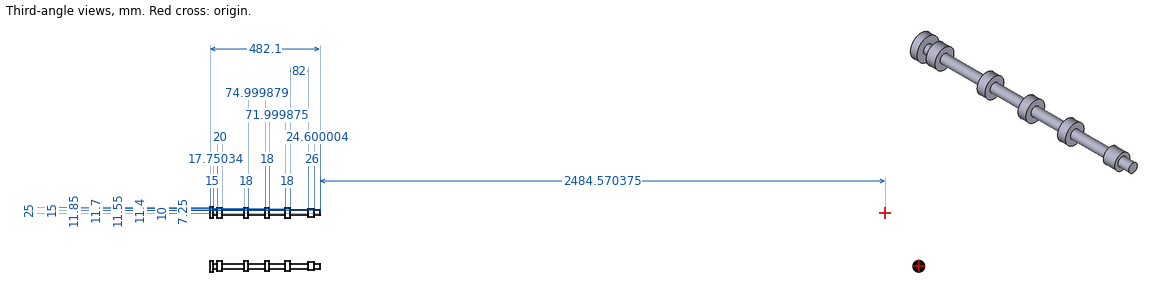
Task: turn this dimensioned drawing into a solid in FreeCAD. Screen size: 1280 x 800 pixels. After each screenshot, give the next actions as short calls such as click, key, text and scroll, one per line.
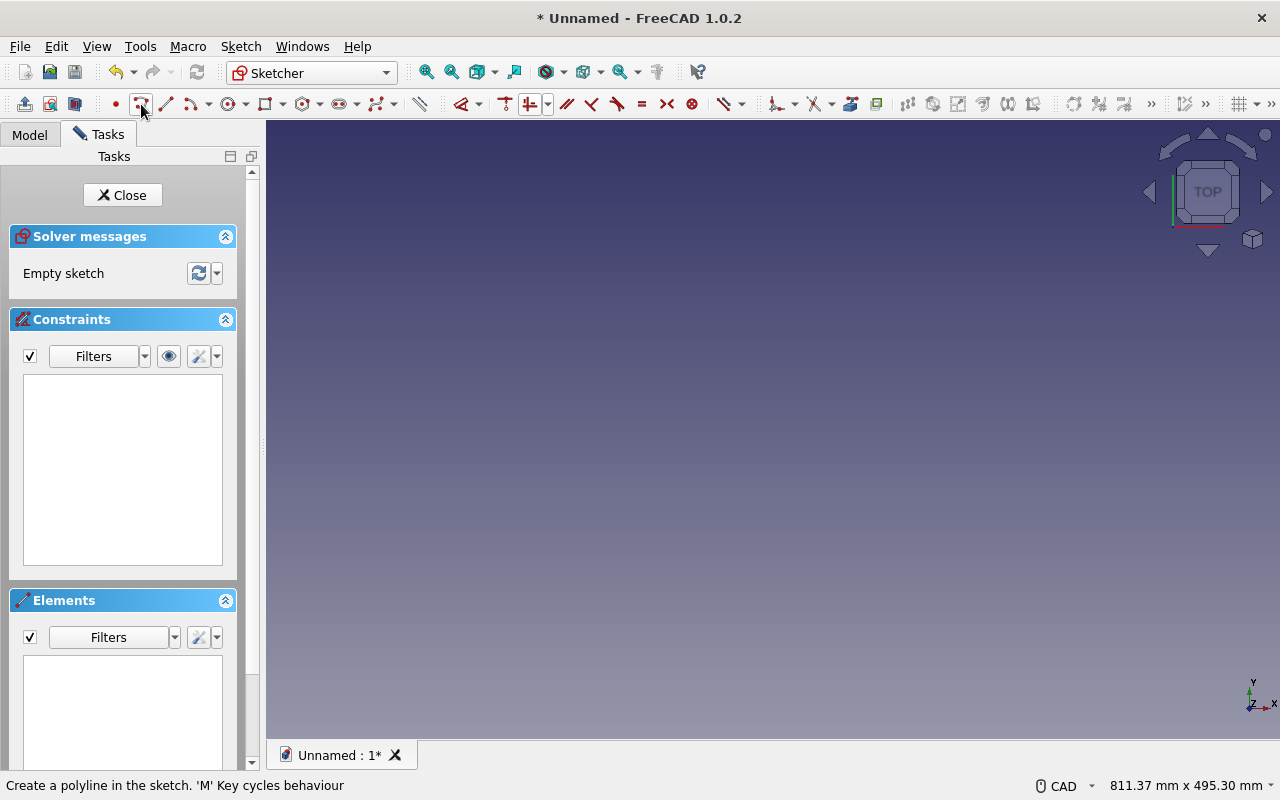
click(995, 430)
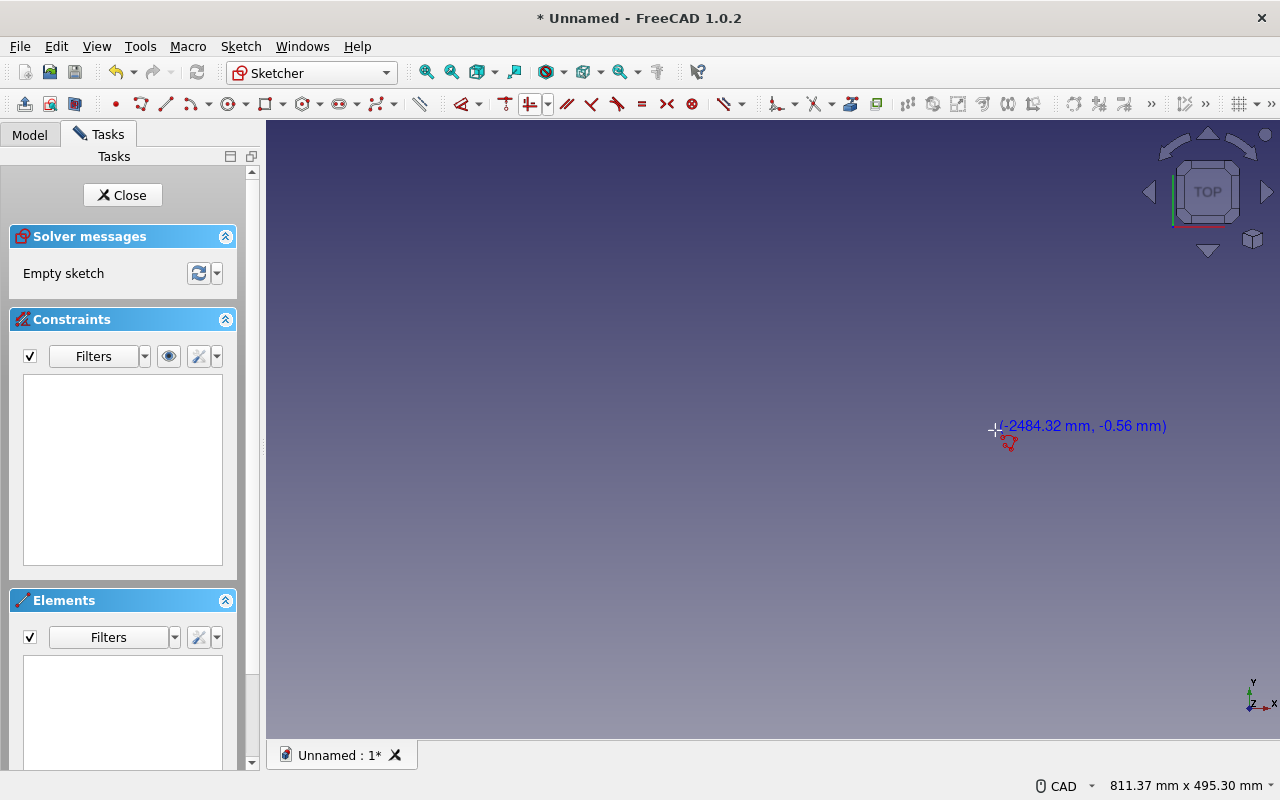
scroll(995, 418, up, 2)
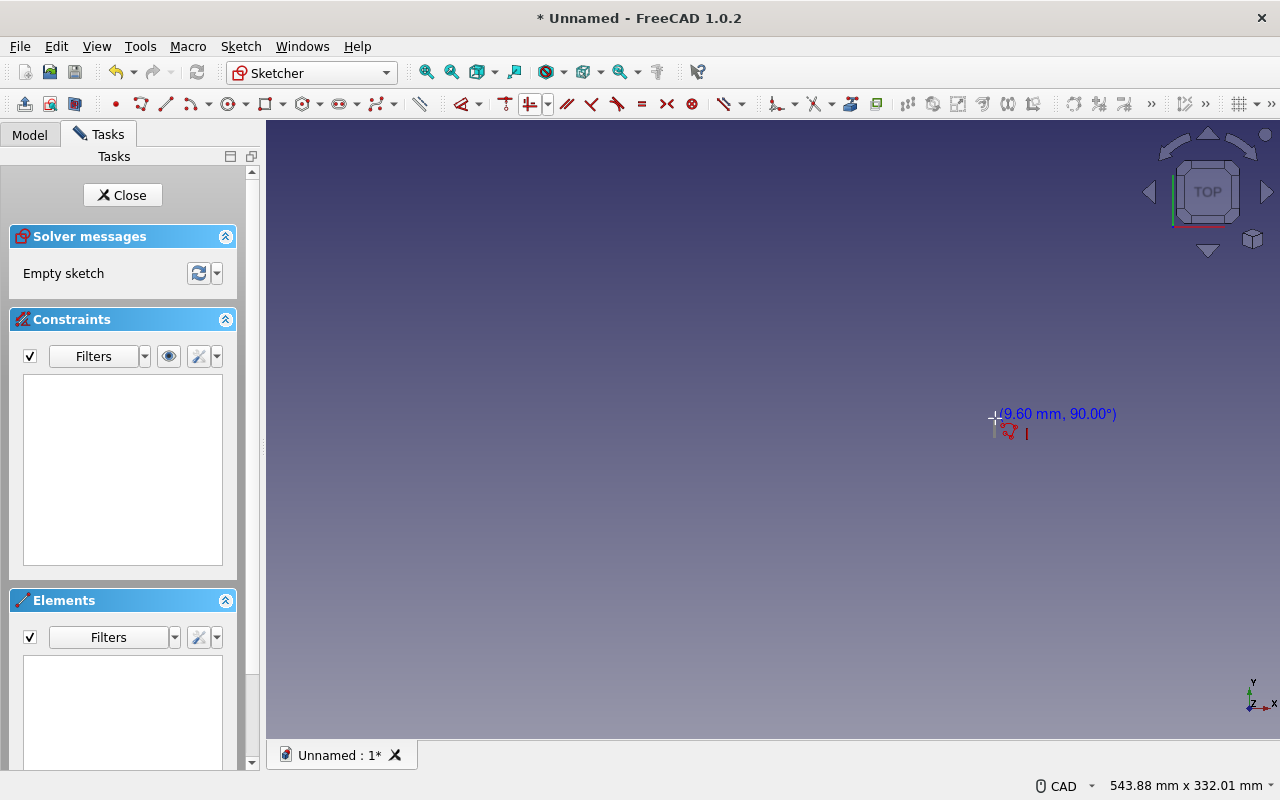
click(995, 417)
click(948, 417)
click(948, 404)
click(900, 404)
click(900, 417)
click(747, 417)
click(747, 396)
click(713, 396)
click(713, 417)
click(579, 417)
click(579, 396)
click(546, 396)
click(546, 417)
click(406, 417)
click(406, 396)
click(372, 396)
click(372, 417)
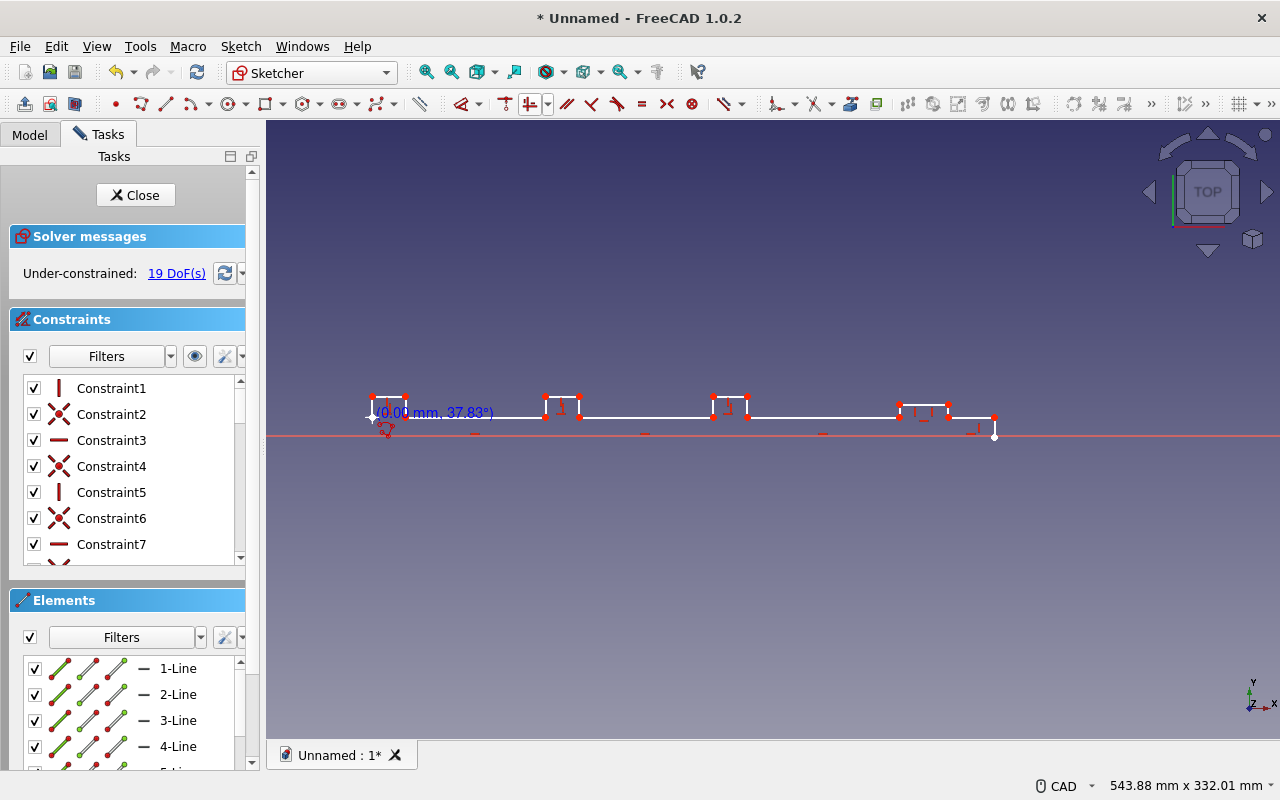
scroll(1029, 463, down, 2)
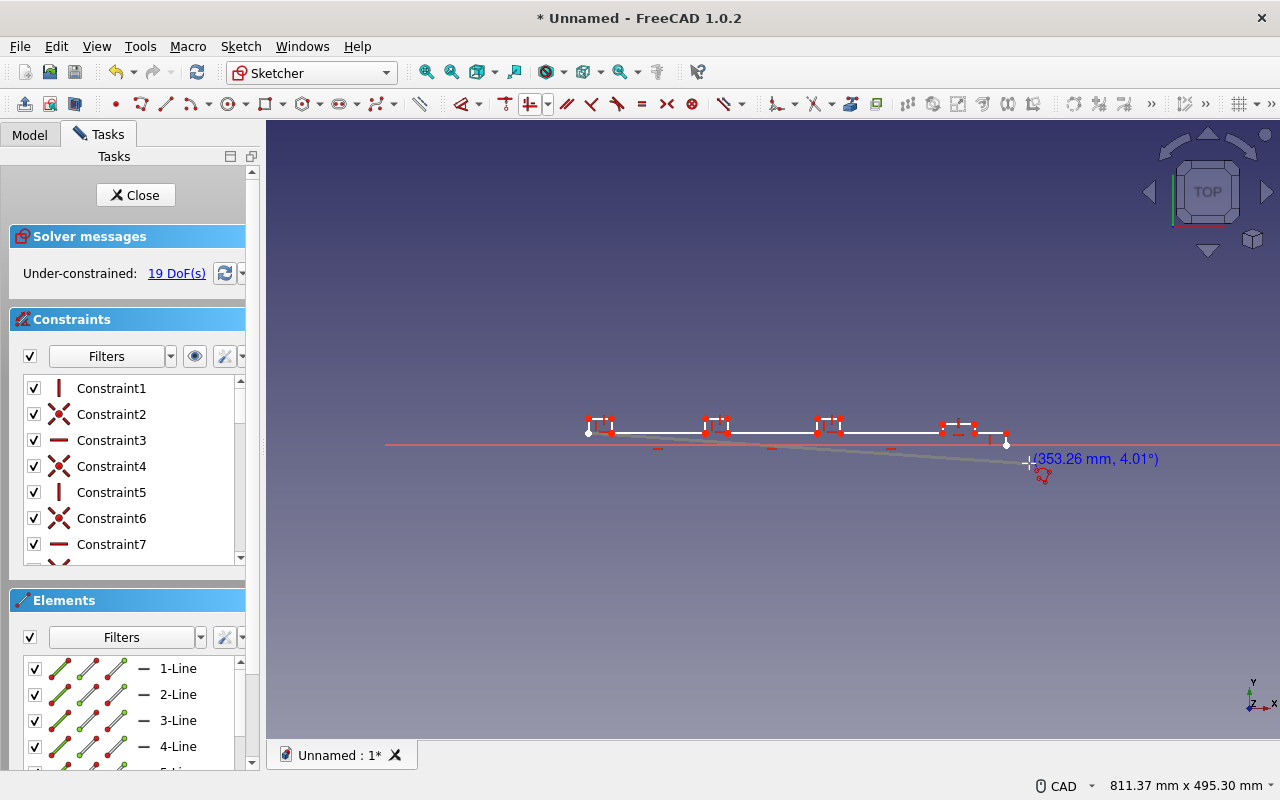
scroll(469, 433, up, 2)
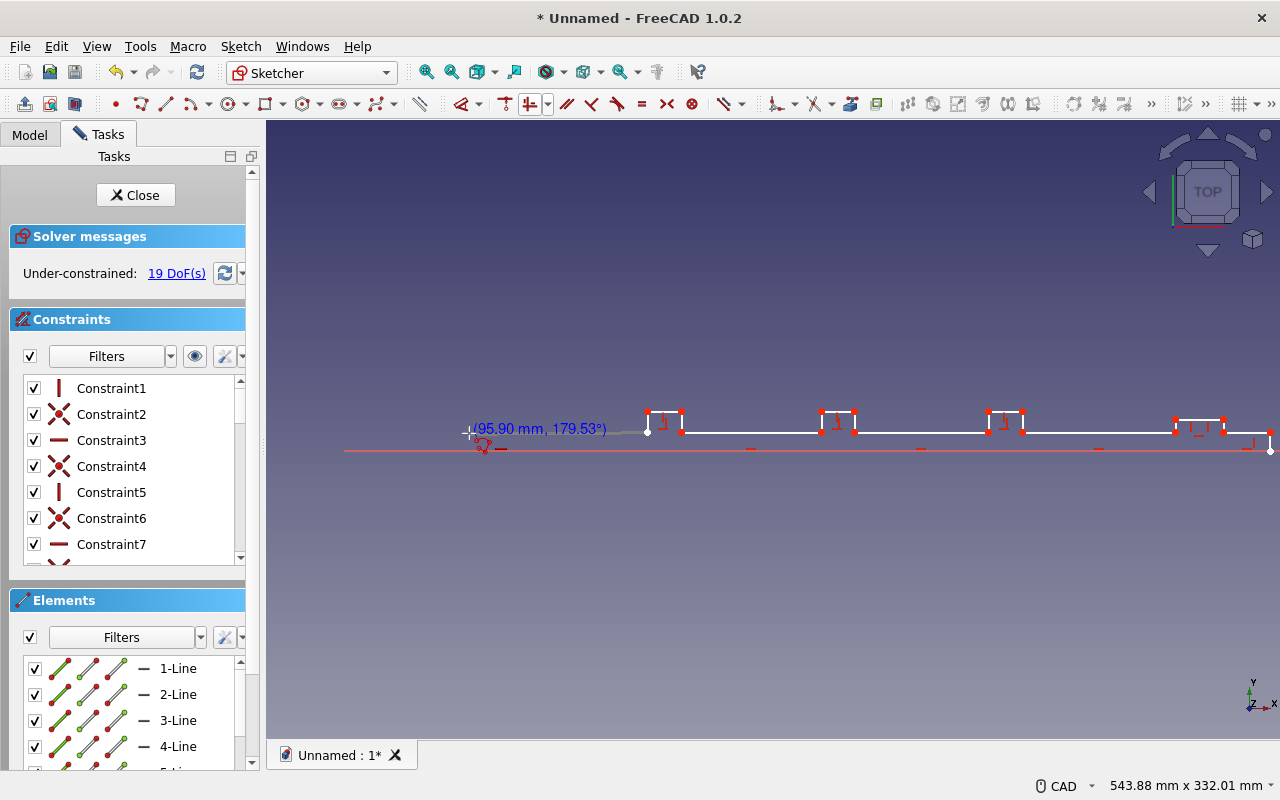
click(469, 432)
click(469, 410)
click(432, 410)
click(432, 432)
click(399, 432)
click(399, 404)
click(371, 404)
click(371, 442)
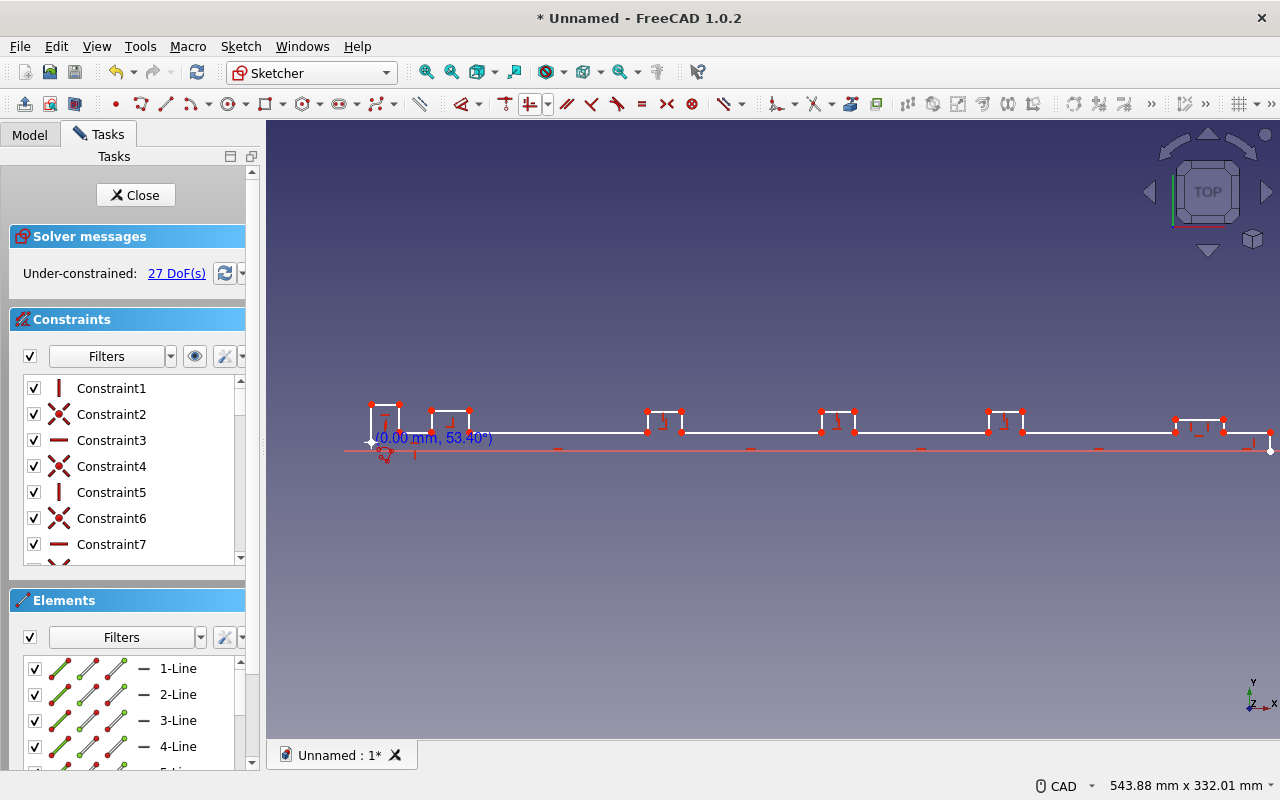
scroll(469, 433, down, 2)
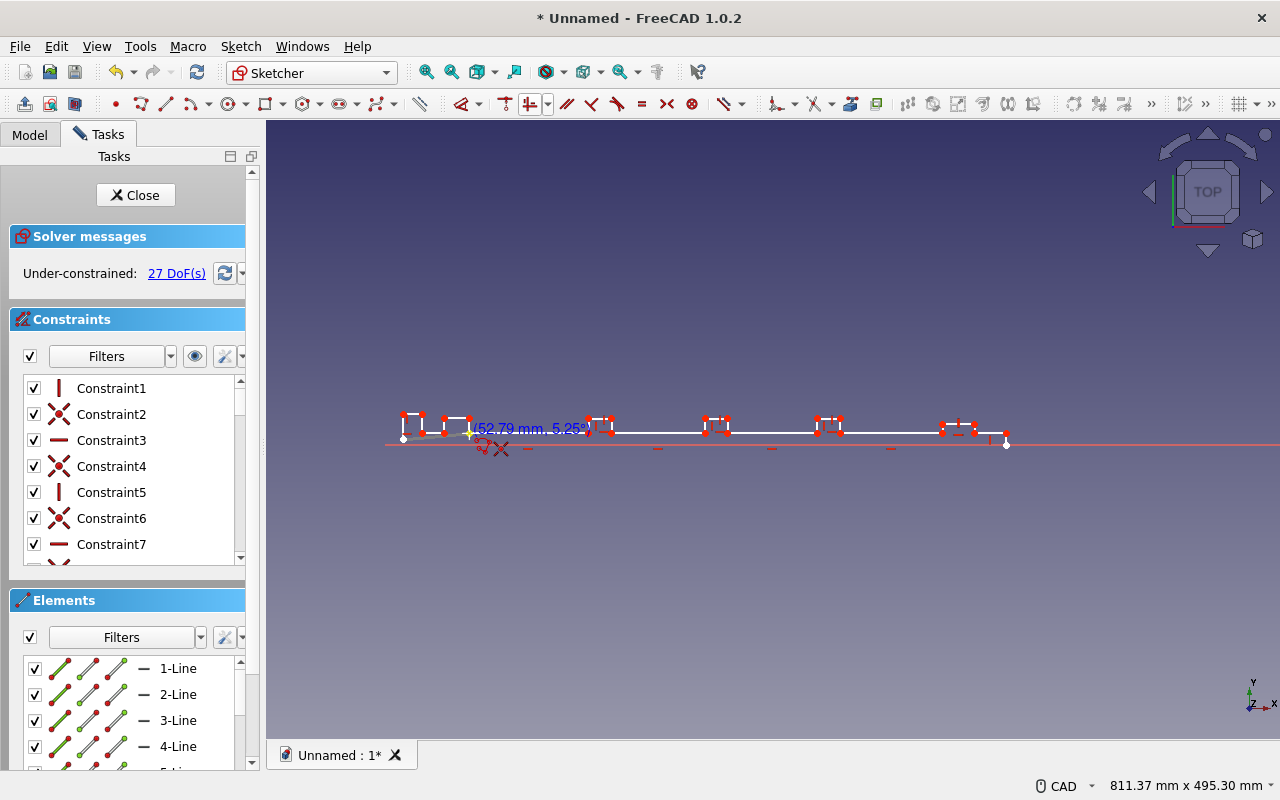
scroll(1006, 445, up, 5)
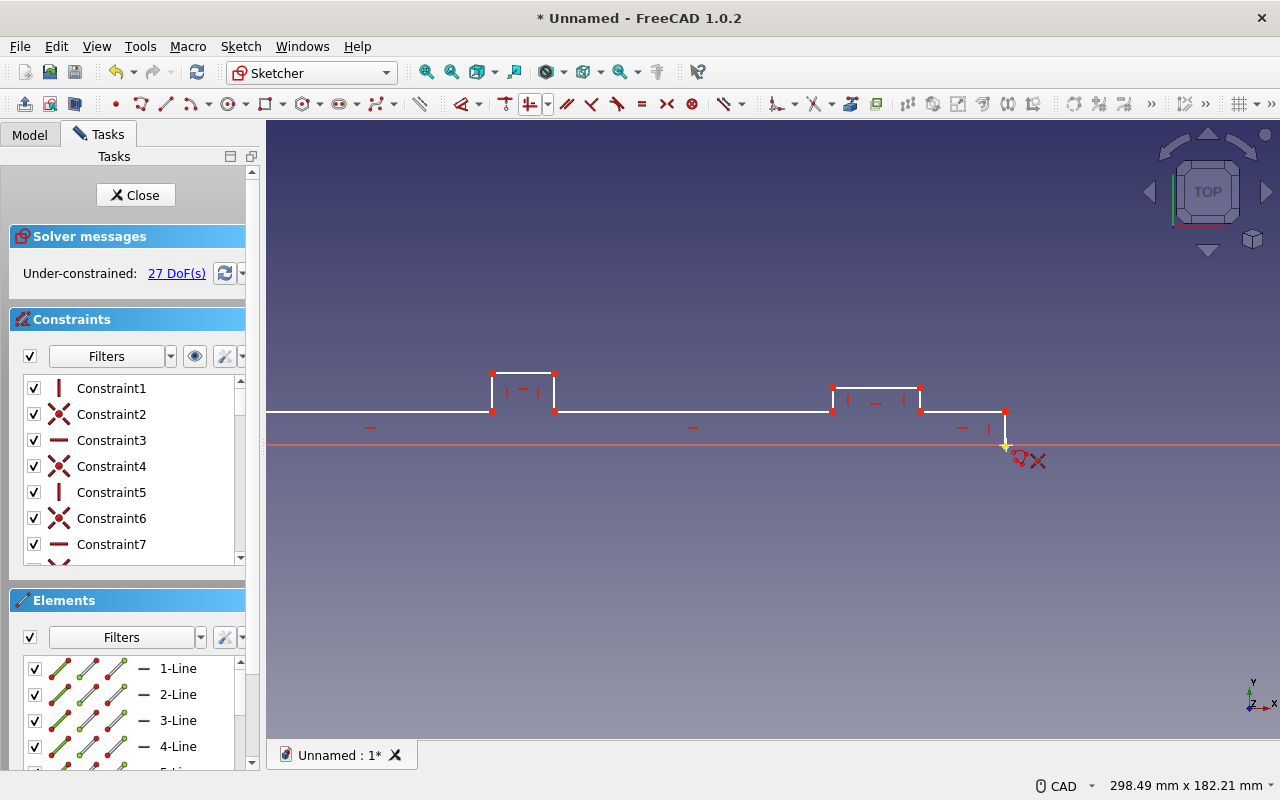
click(1005, 446)
key(Escape)
key(Escape)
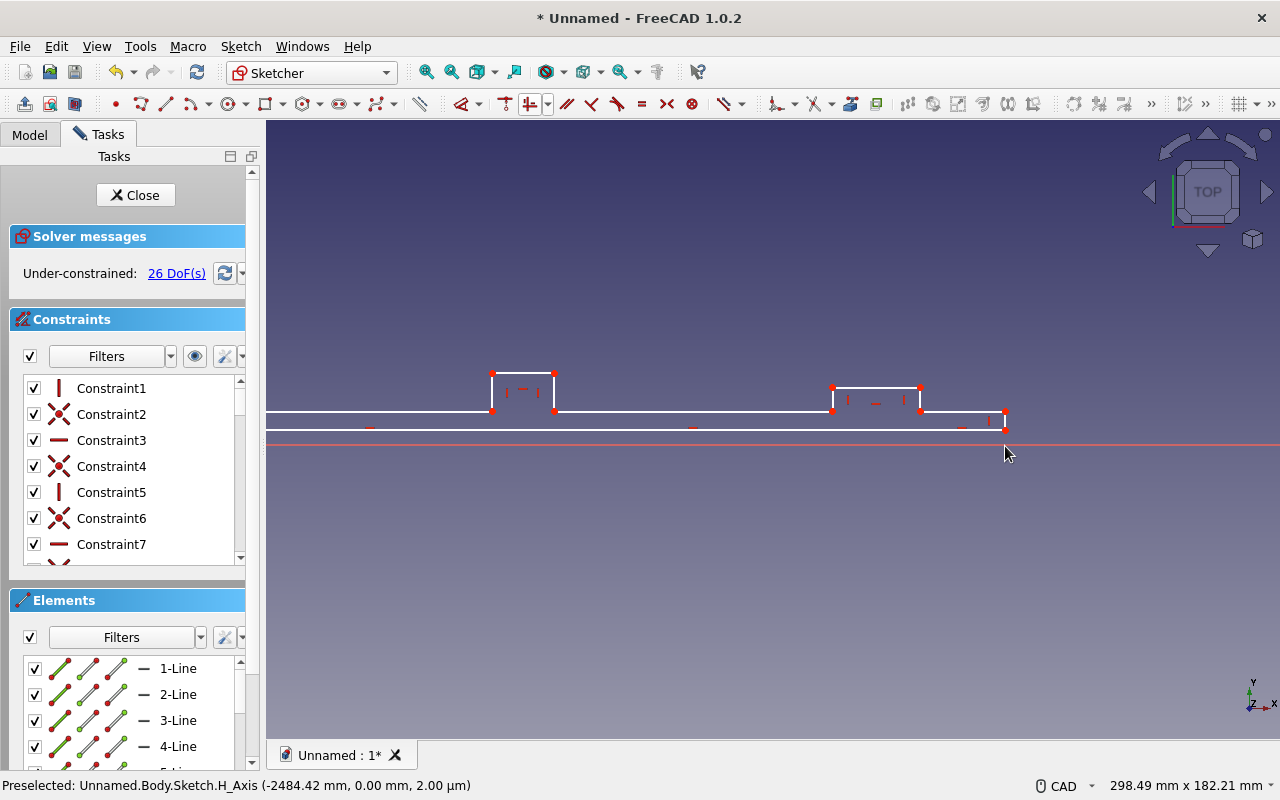
click(1005, 430)